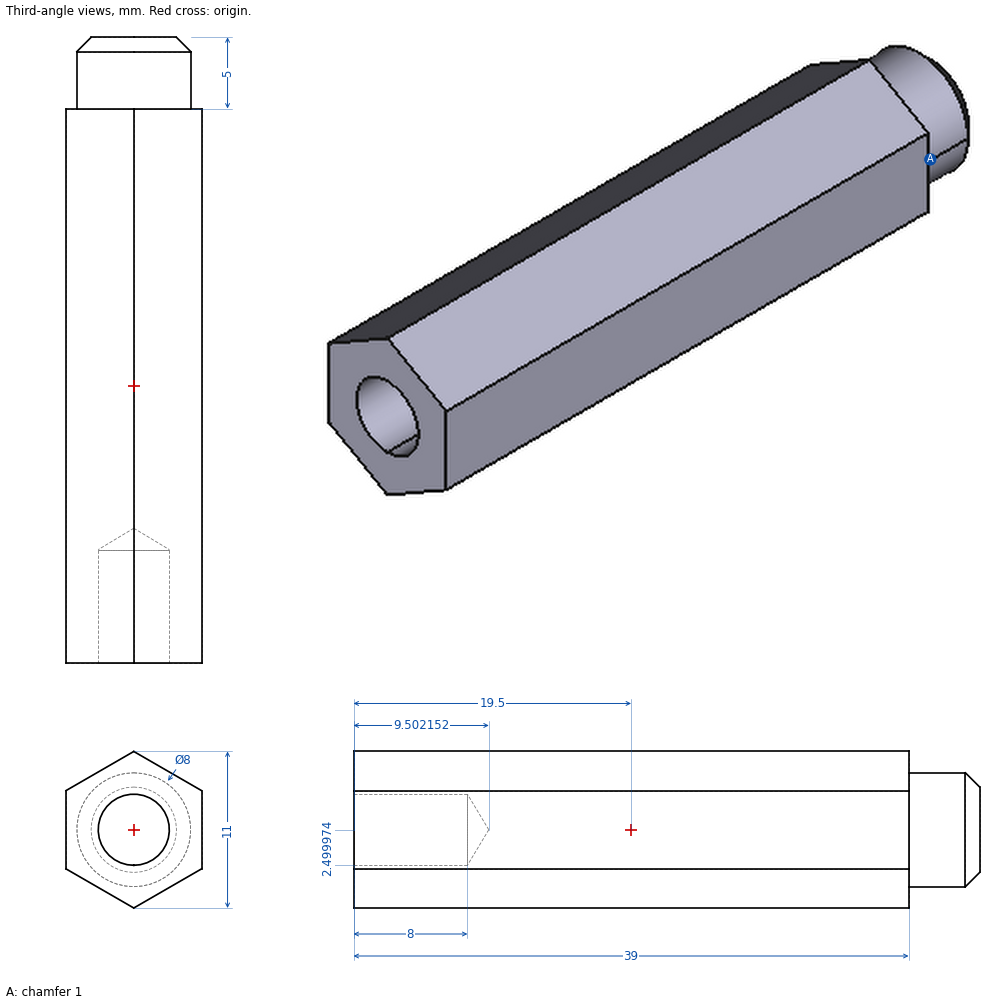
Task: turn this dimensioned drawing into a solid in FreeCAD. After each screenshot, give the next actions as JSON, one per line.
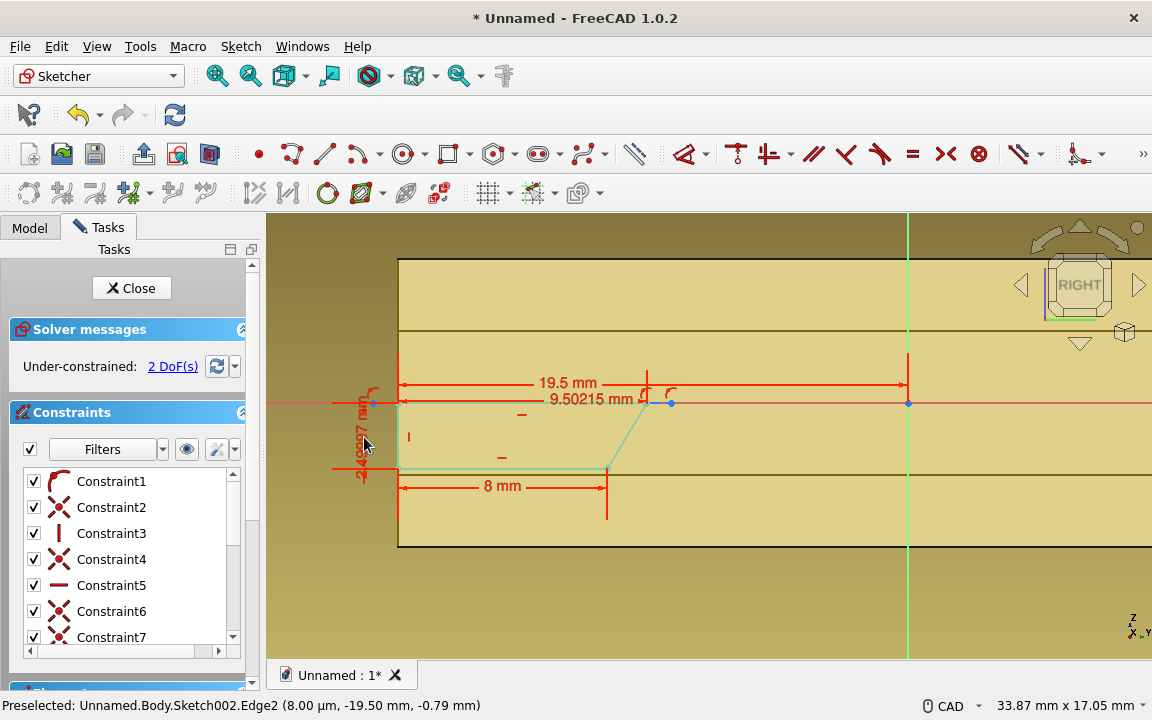
{"action": "left_click", "coordinate": [132, 288]}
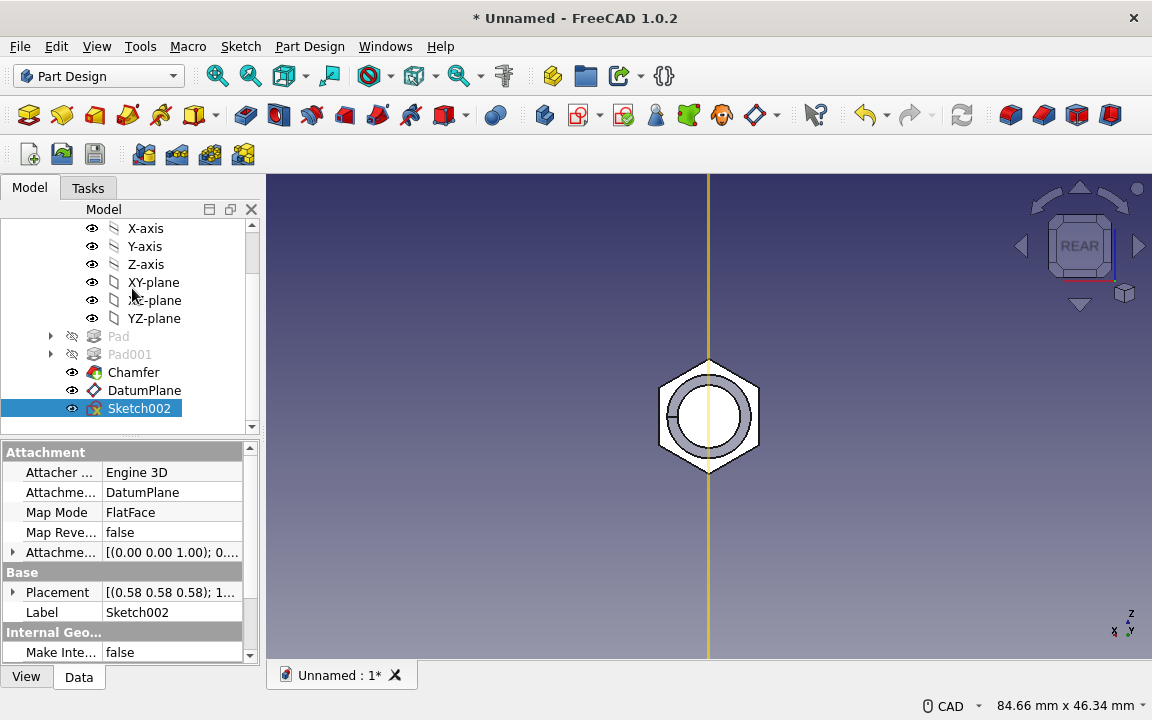
{"action": "left_click", "coordinate": [312, 116]}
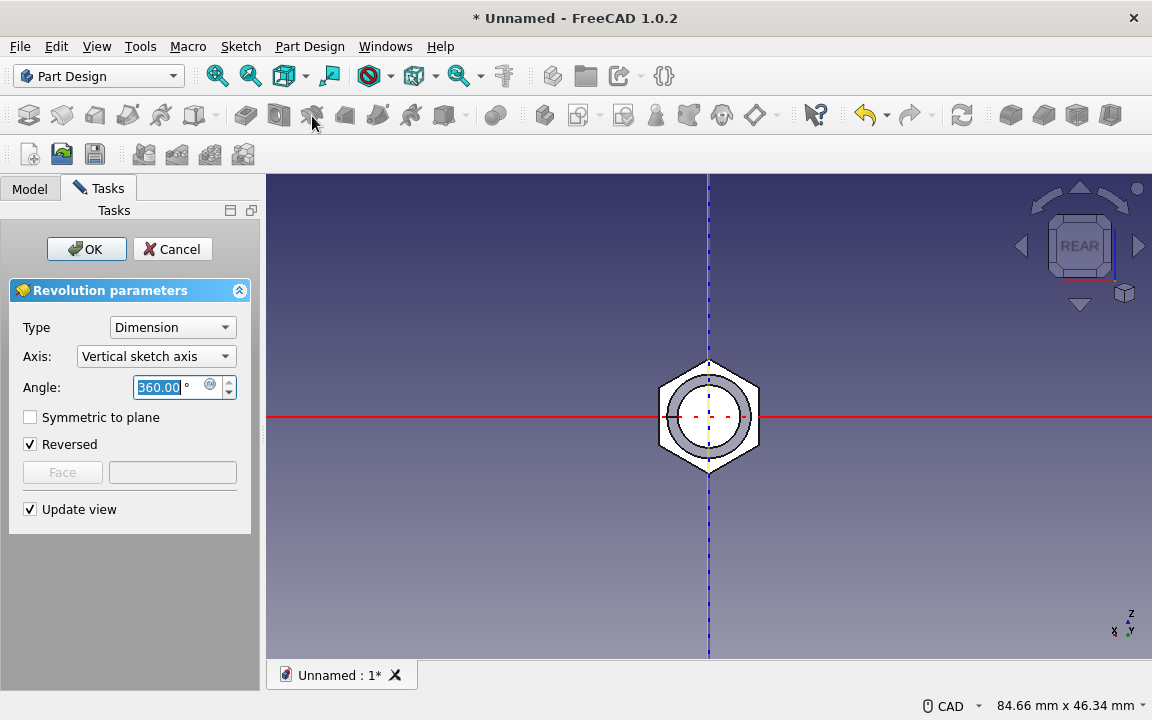
{"action": "left_click", "coordinate": [157, 356]}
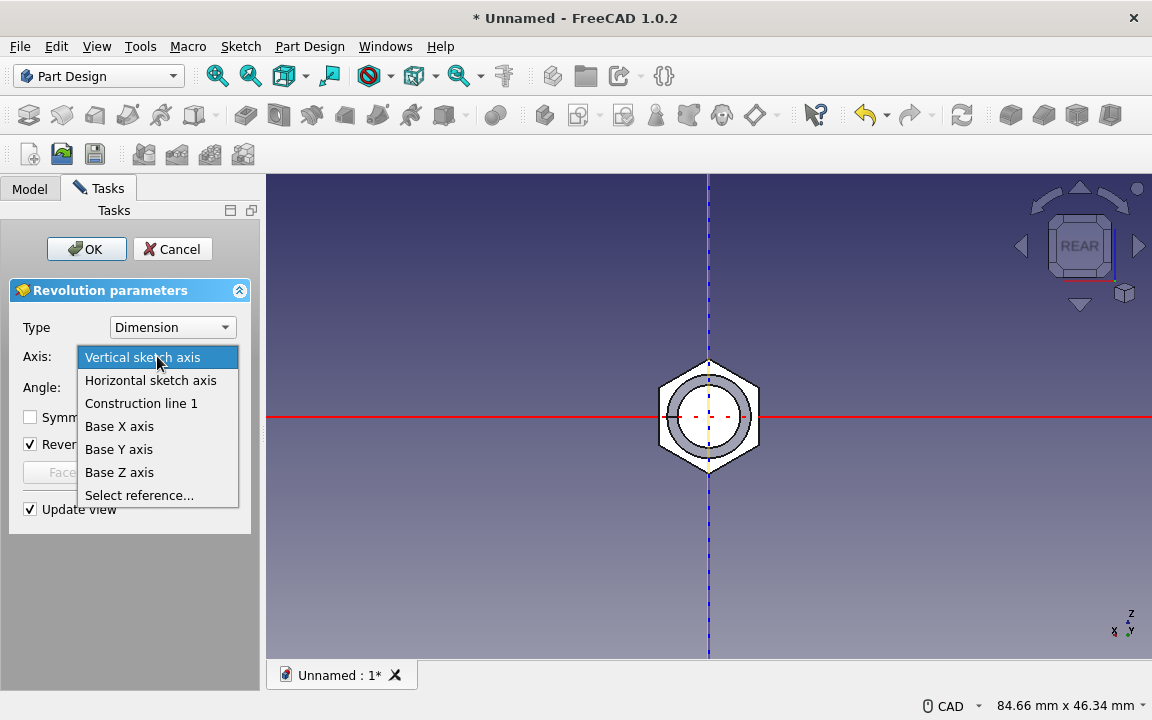
{"action": "left_click", "coordinate": [156, 404]}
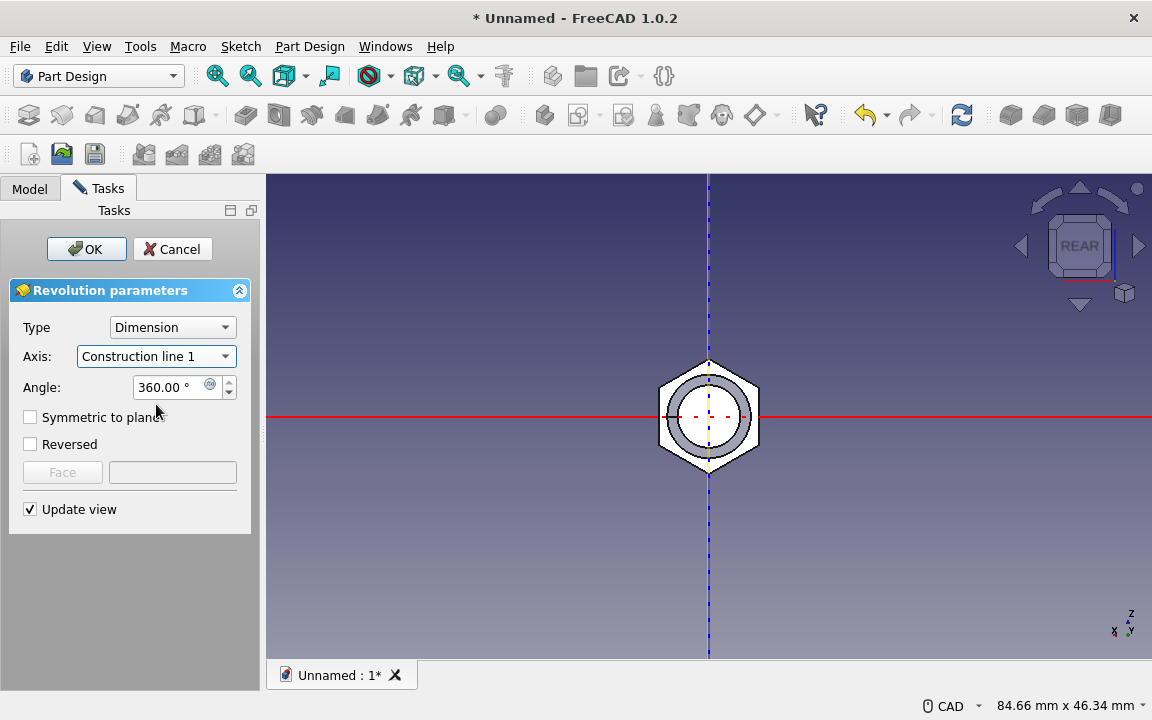
{"action": "left_click", "coordinate": [87, 249]}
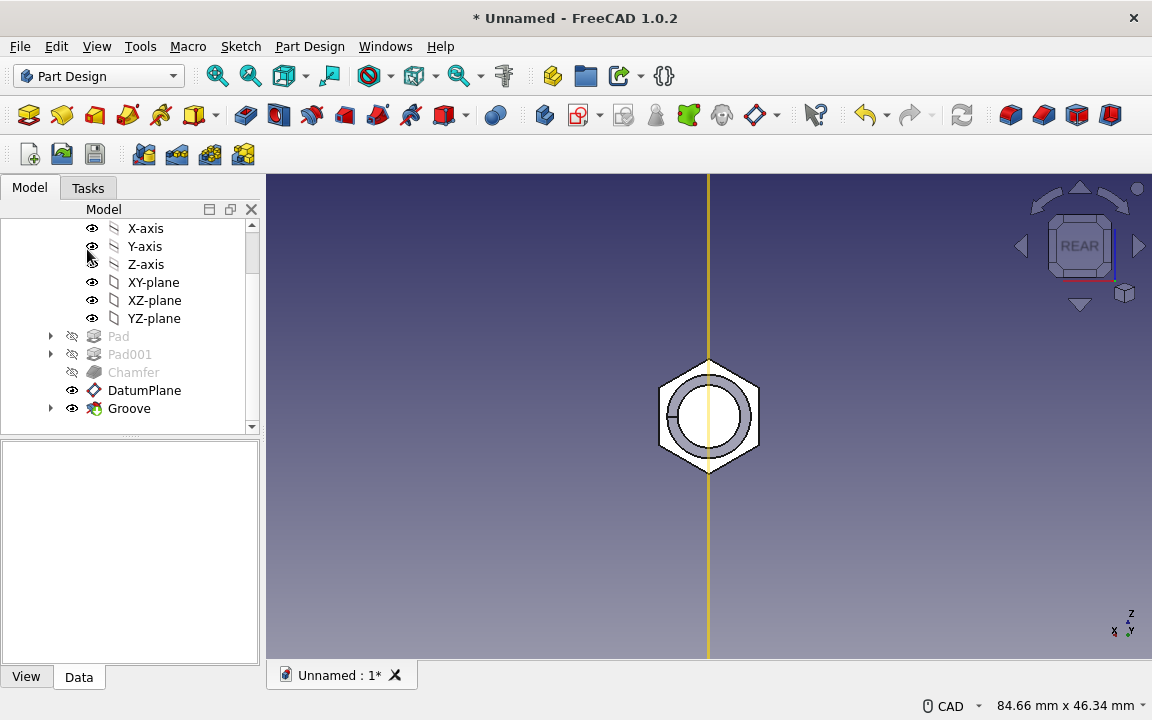
{"action": "left_click", "coordinate": [117, 390]}
{"action": "key", "text": "space"}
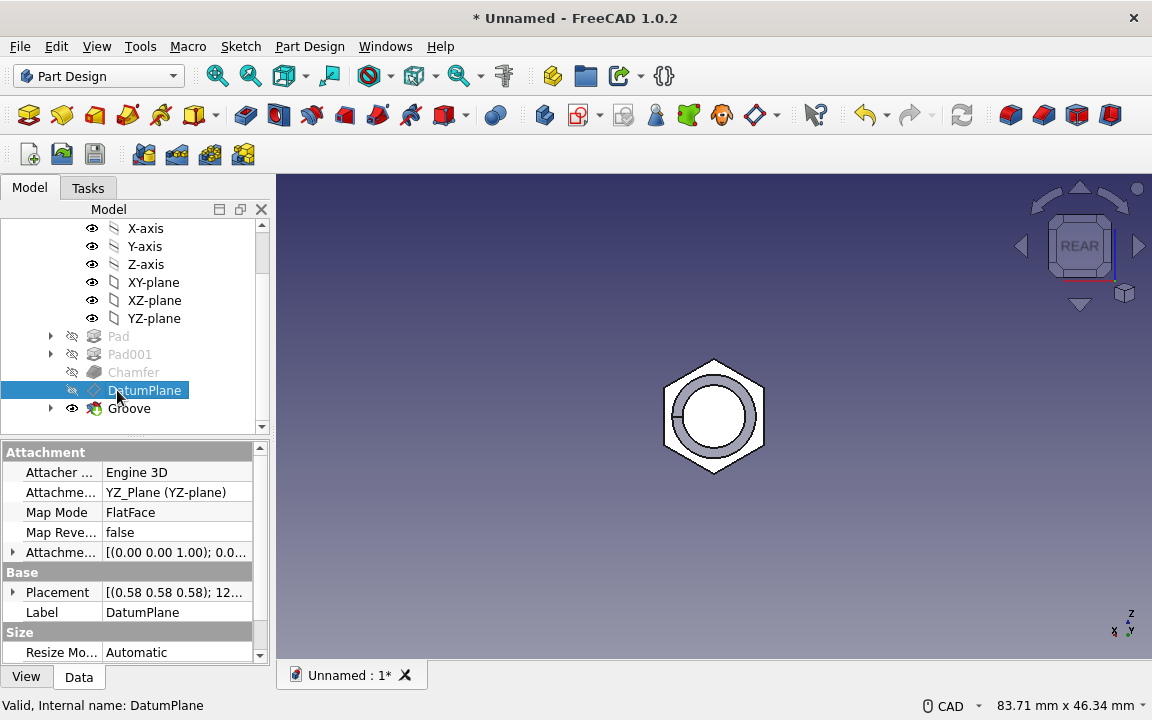
{"action": "key", "text": "0"}